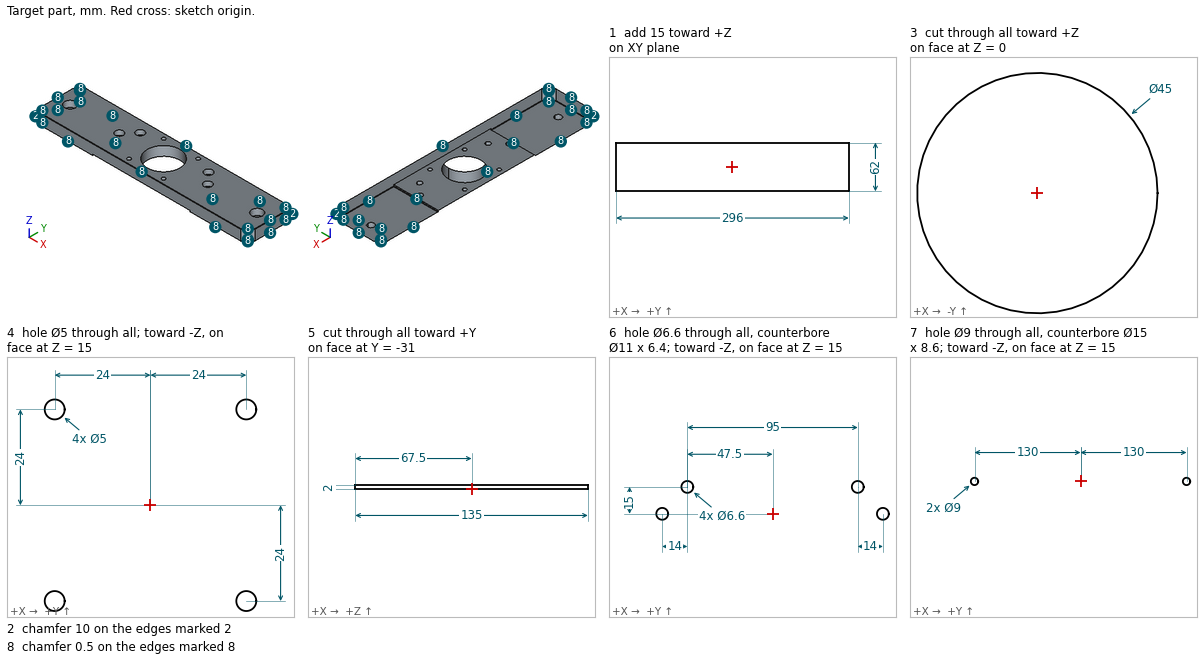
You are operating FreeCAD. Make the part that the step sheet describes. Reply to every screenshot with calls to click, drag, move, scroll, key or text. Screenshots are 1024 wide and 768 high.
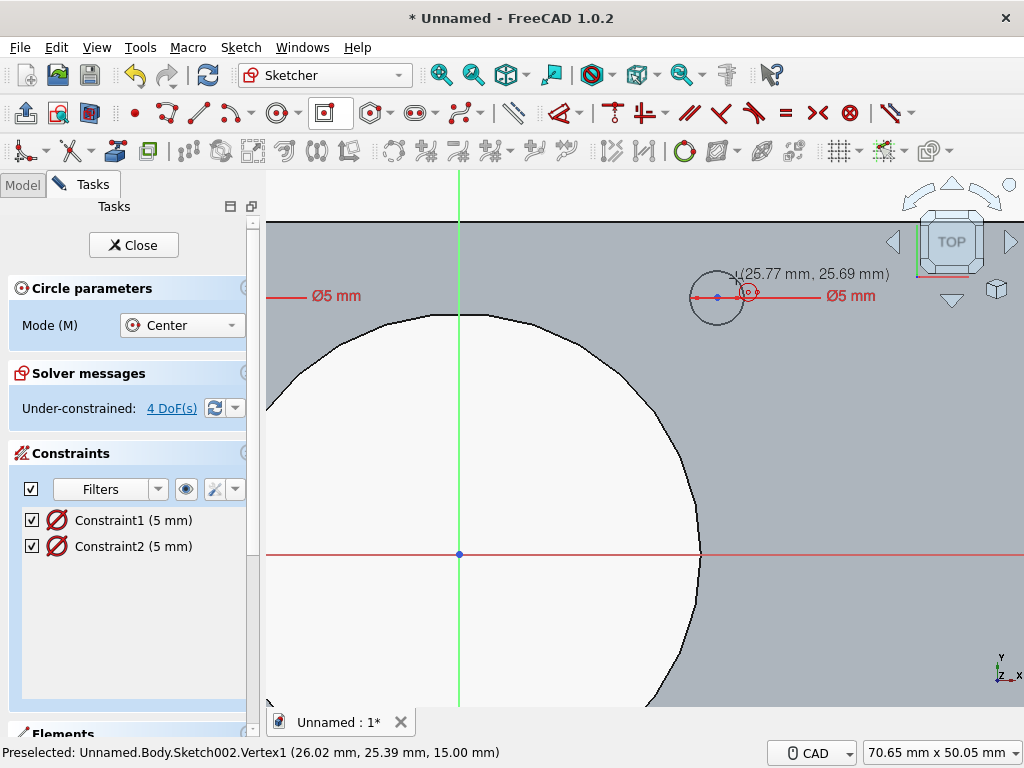
scroll(719, 297, down, 3)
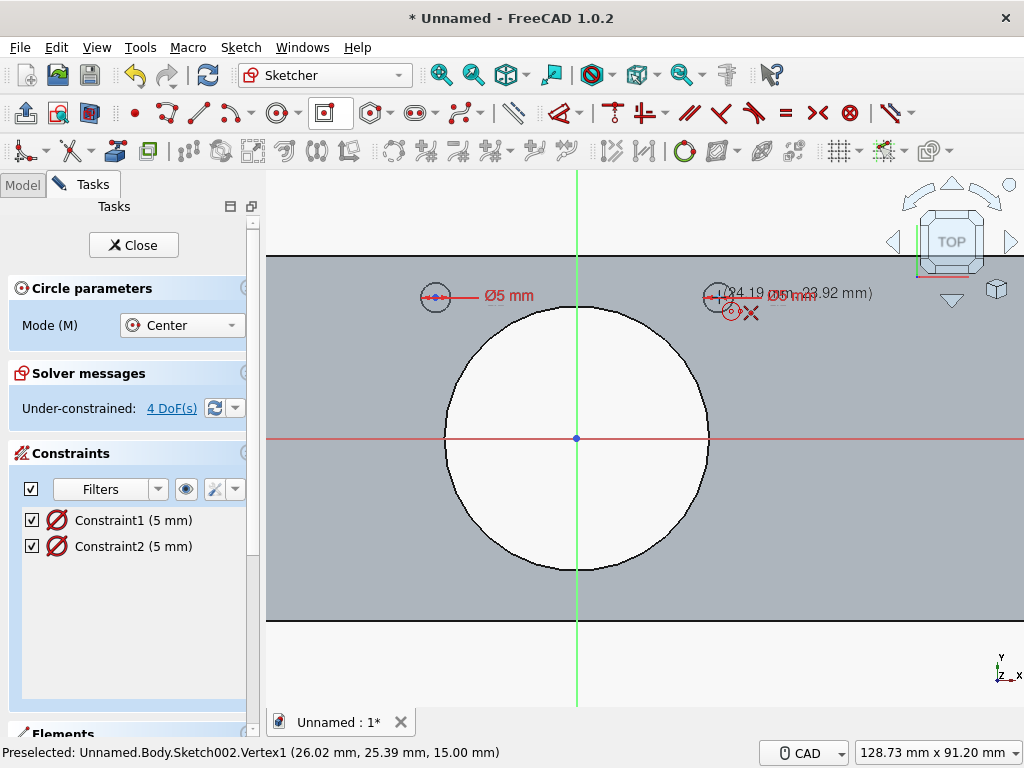
scroll(718, 580, up, 3)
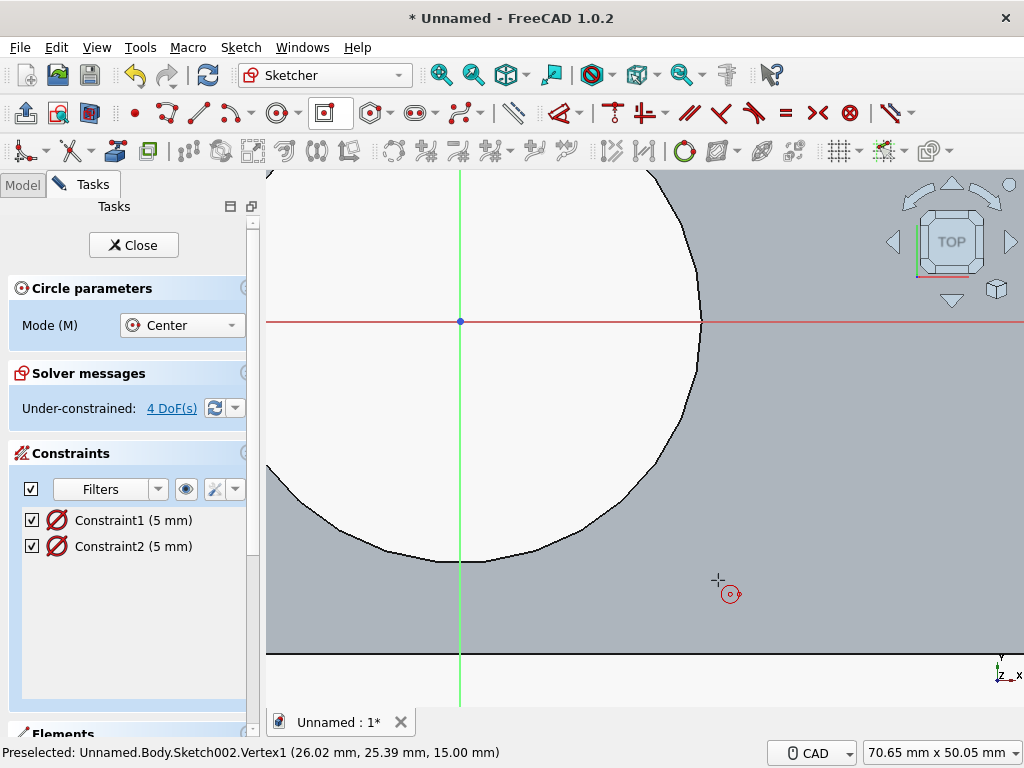
click(718, 579)
move(737, 560)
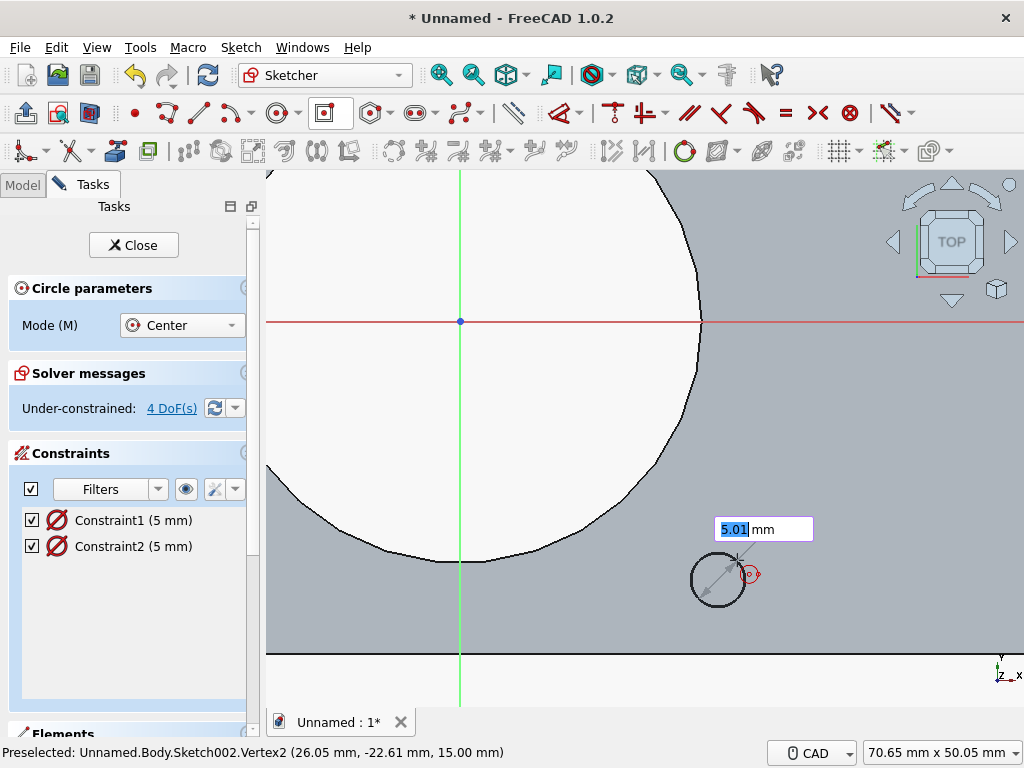
text(5)
key(Return)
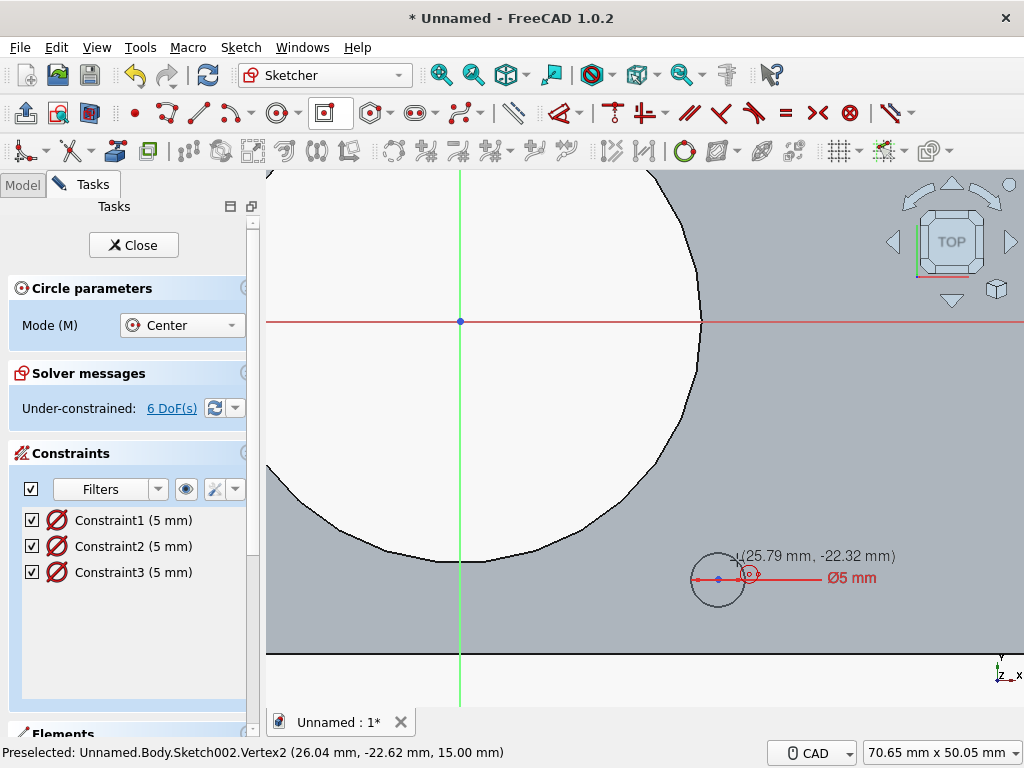
scroll(718, 581, down, 3)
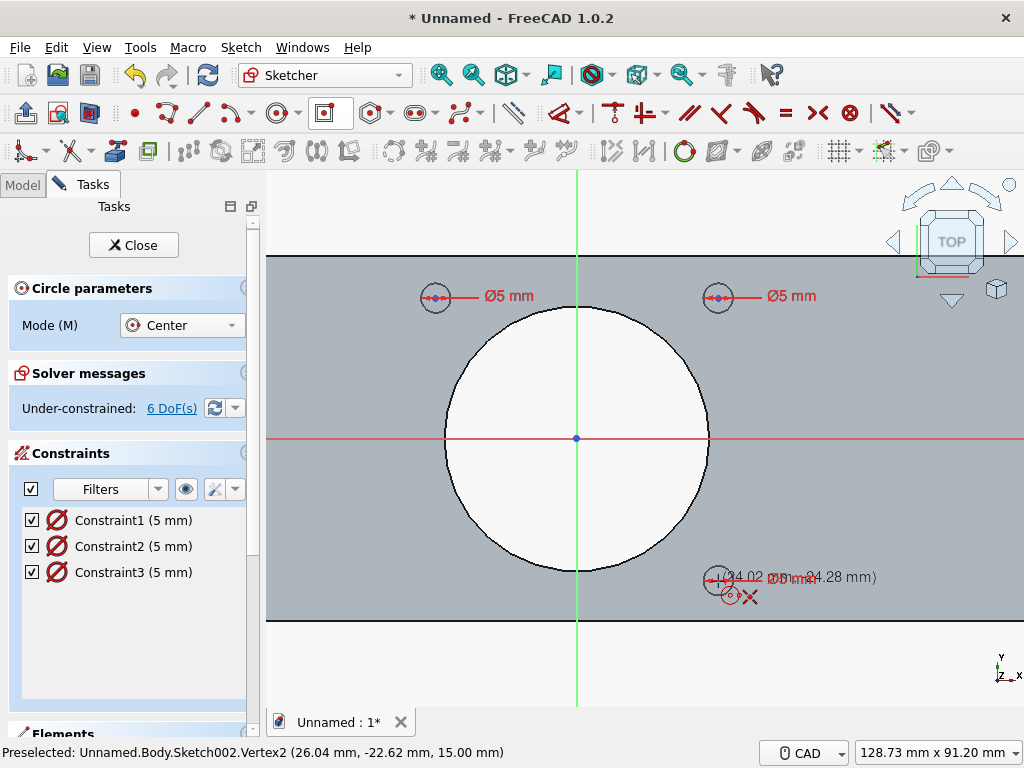
scroll(436, 580, up, 3)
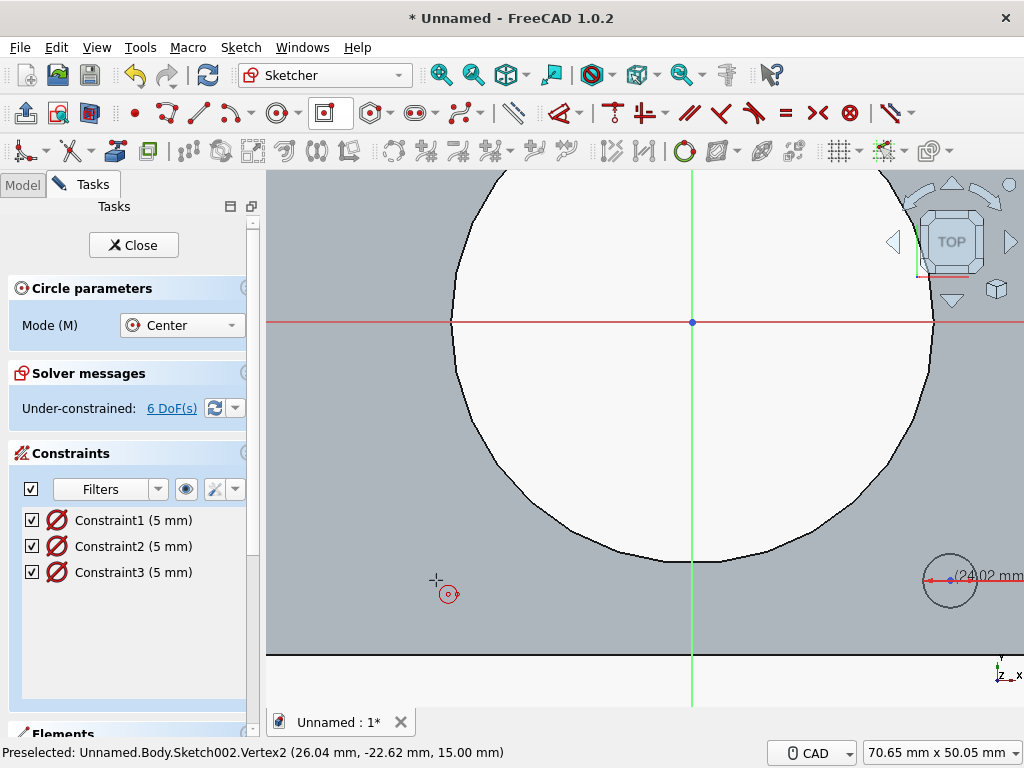
click(435, 580)
move(454, 561)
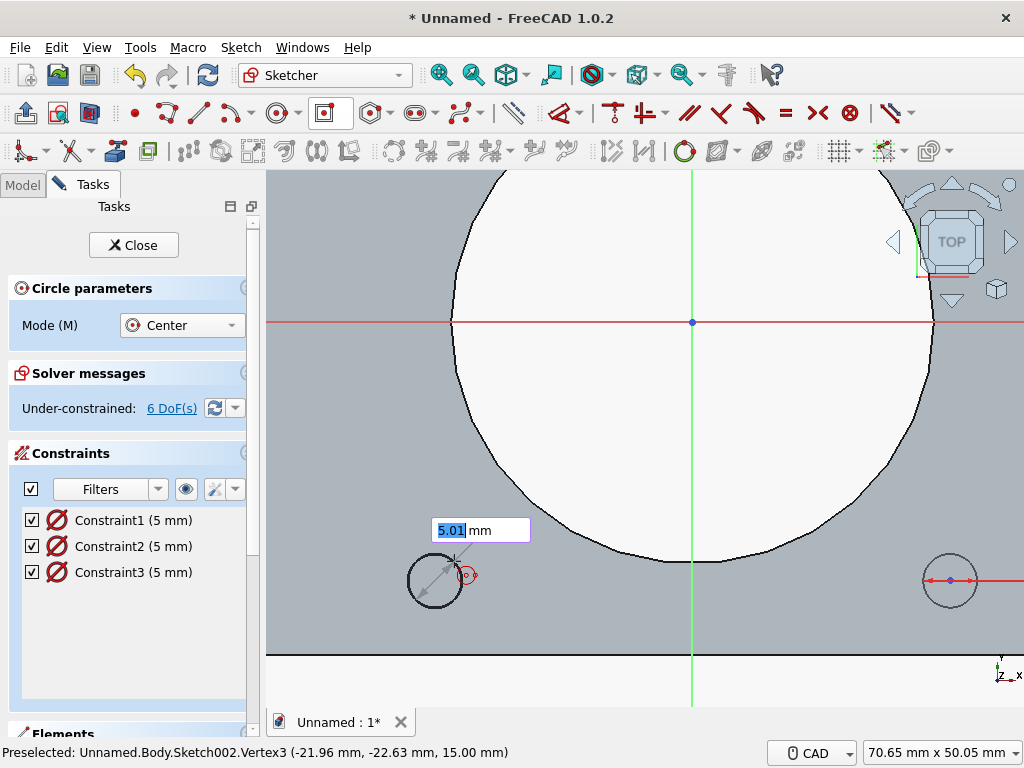
text(5)
key(Return)
key(Escape)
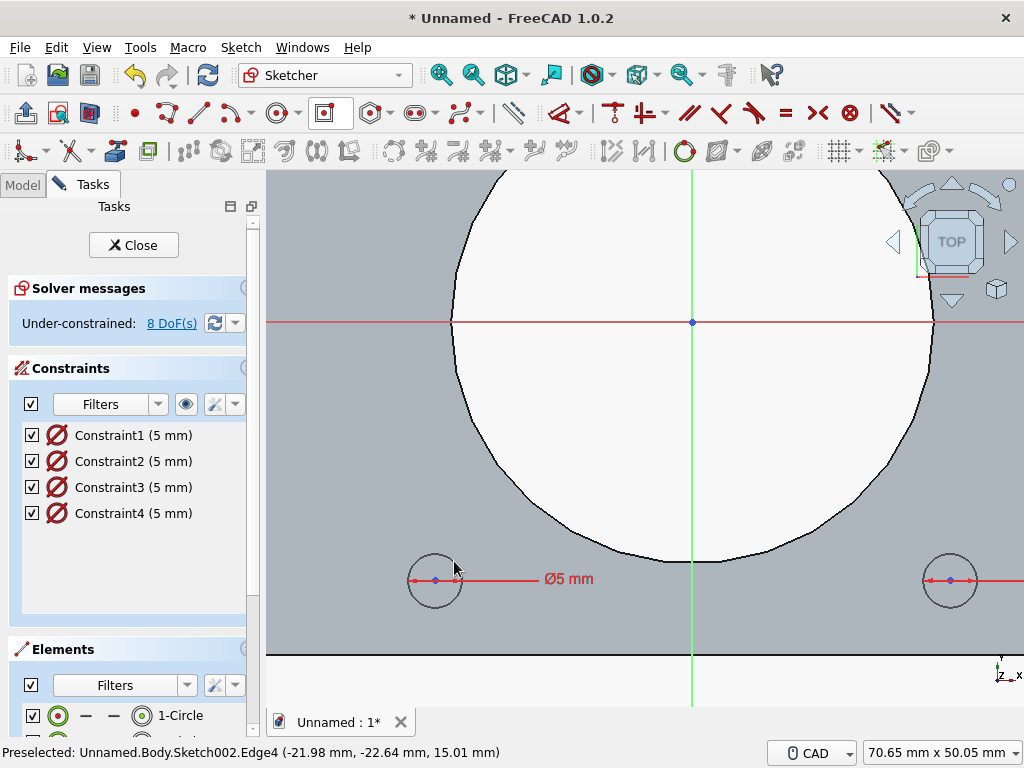
scroll(435, 580, down, 3)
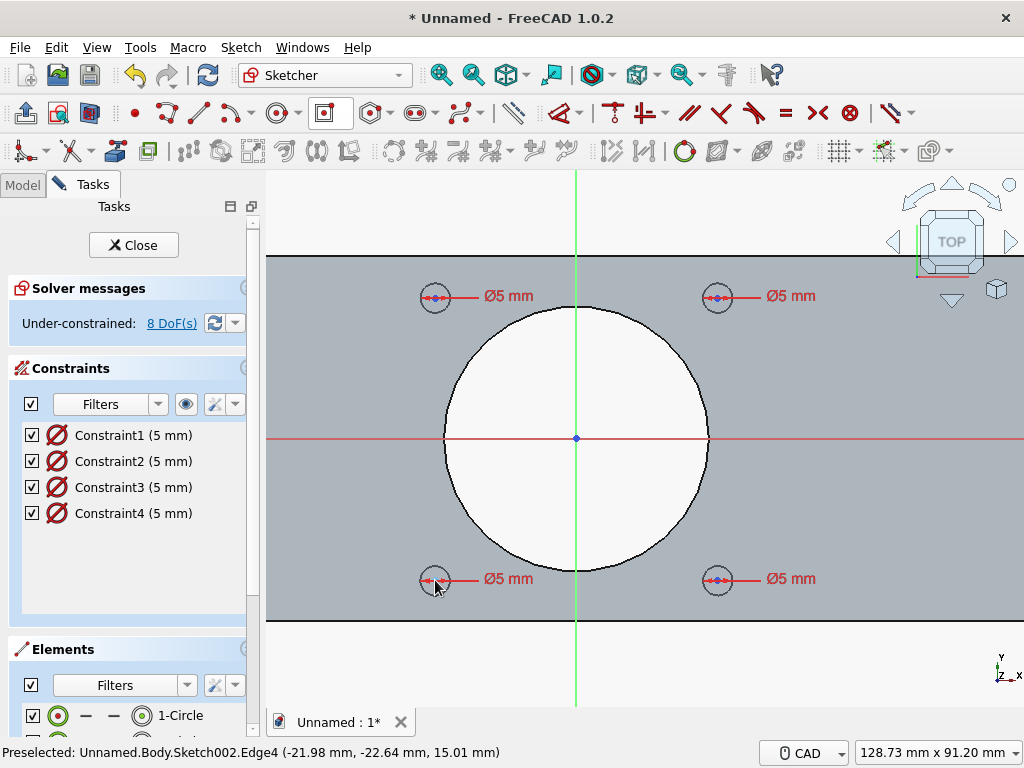
click(435, 298)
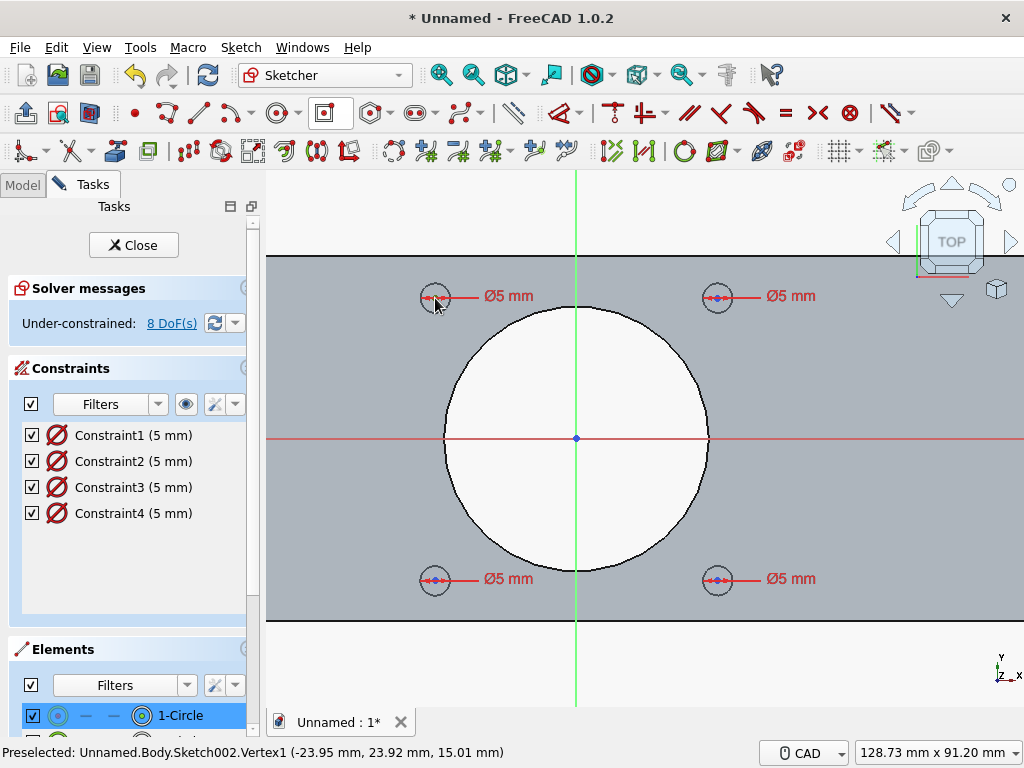
click(718, 298)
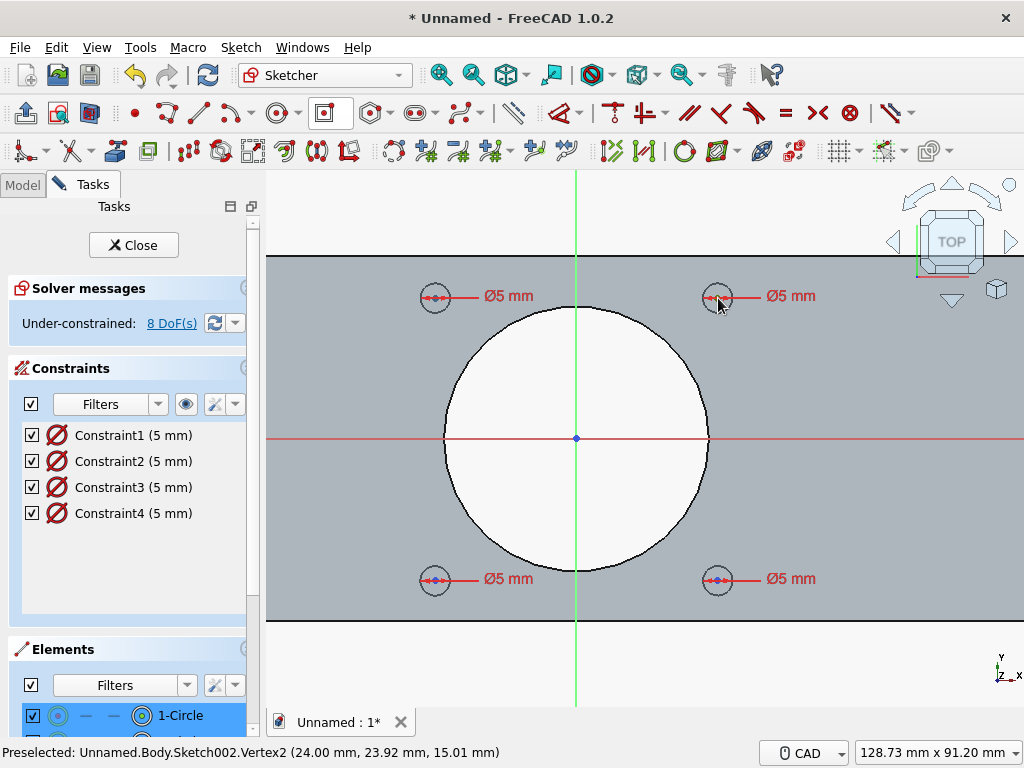
click(668, 114)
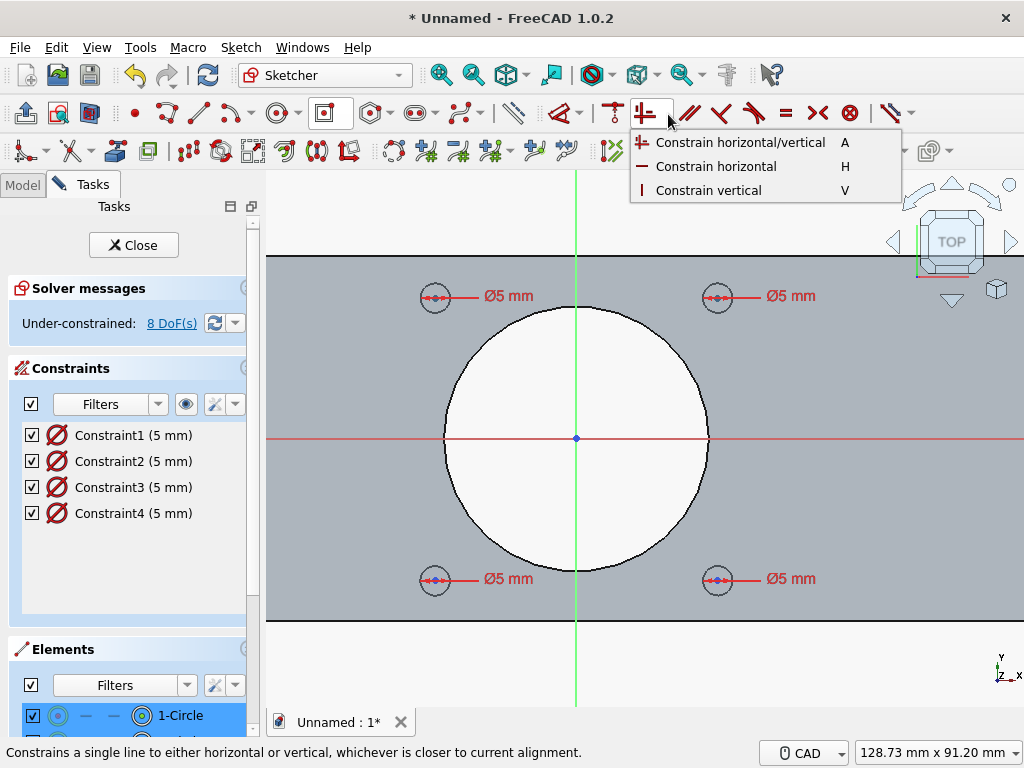
click(766, 166)